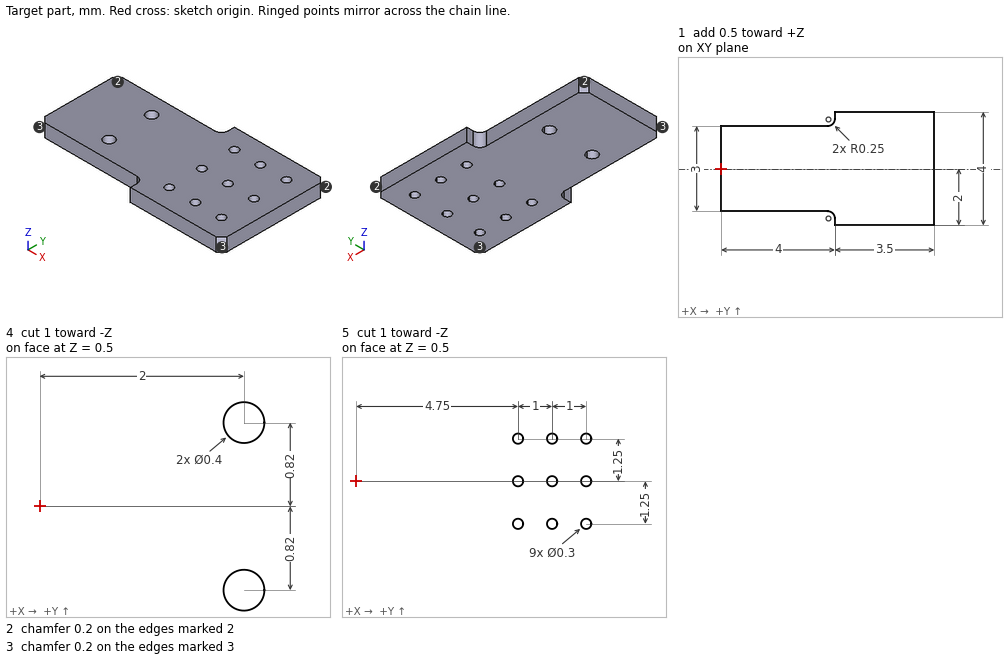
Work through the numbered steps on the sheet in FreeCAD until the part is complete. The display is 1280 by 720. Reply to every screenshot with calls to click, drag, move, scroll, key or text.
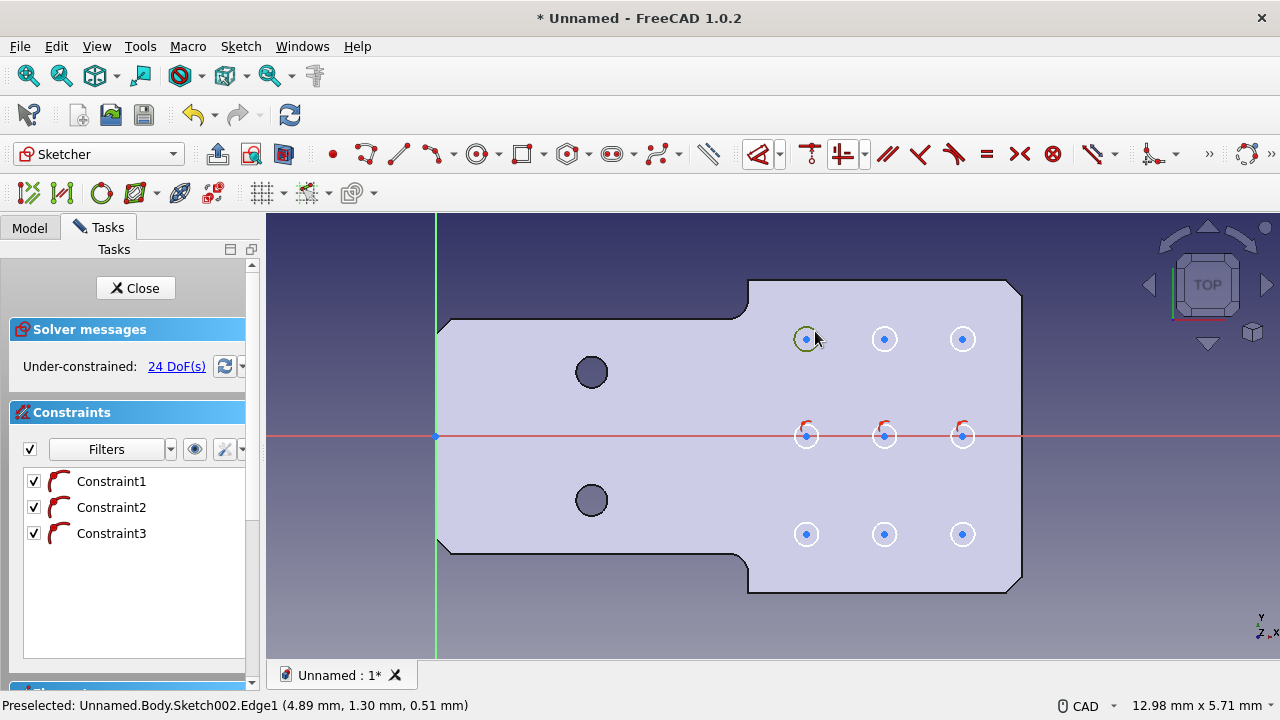
click(893, 331)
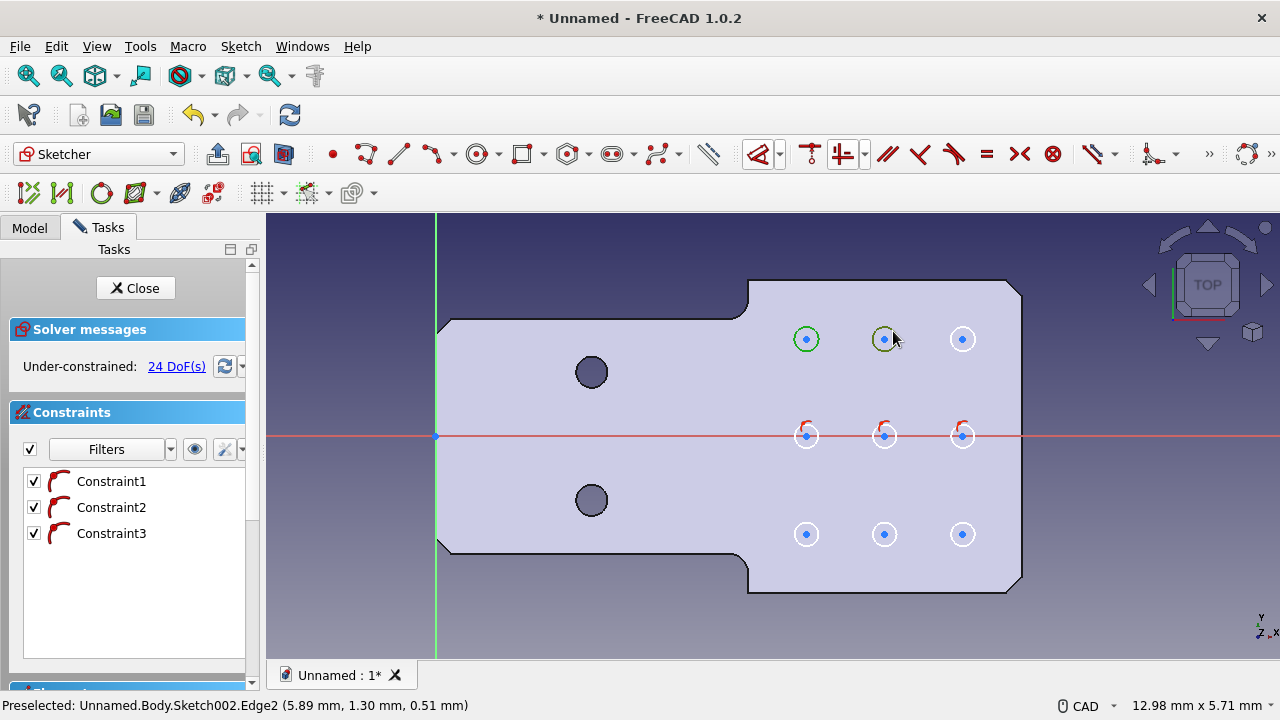
click(971, 331)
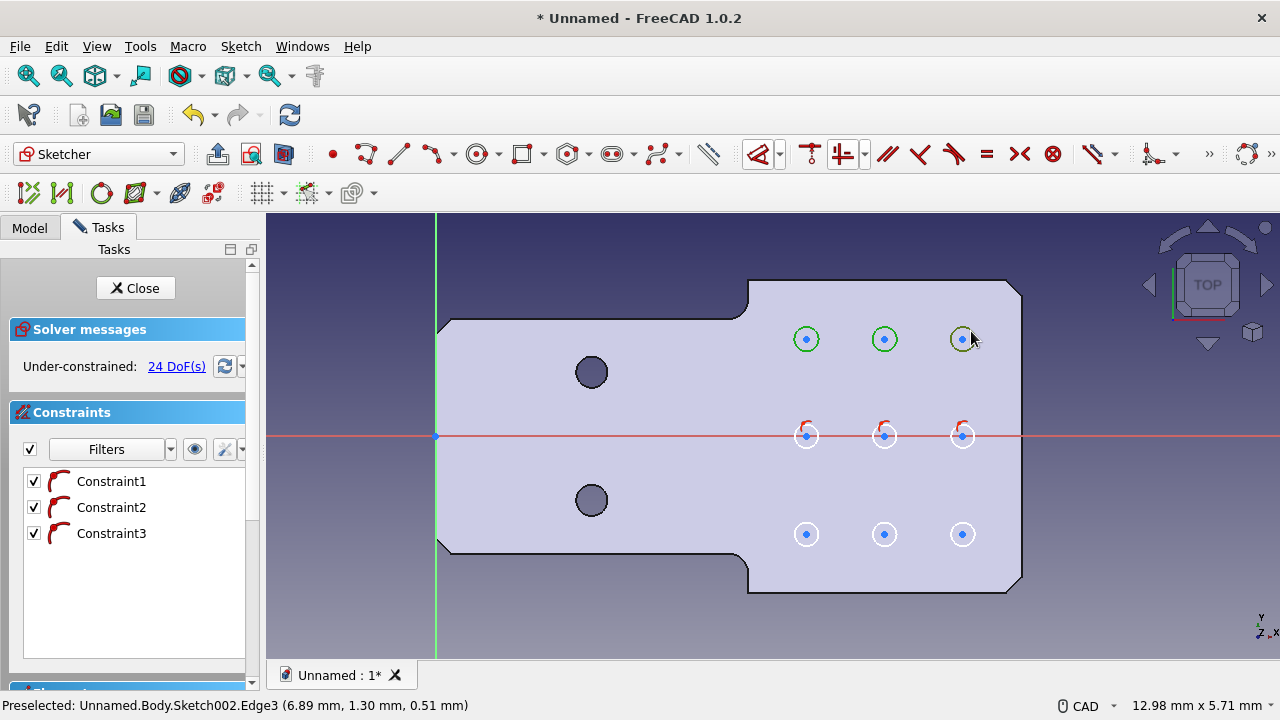
click(951, 436)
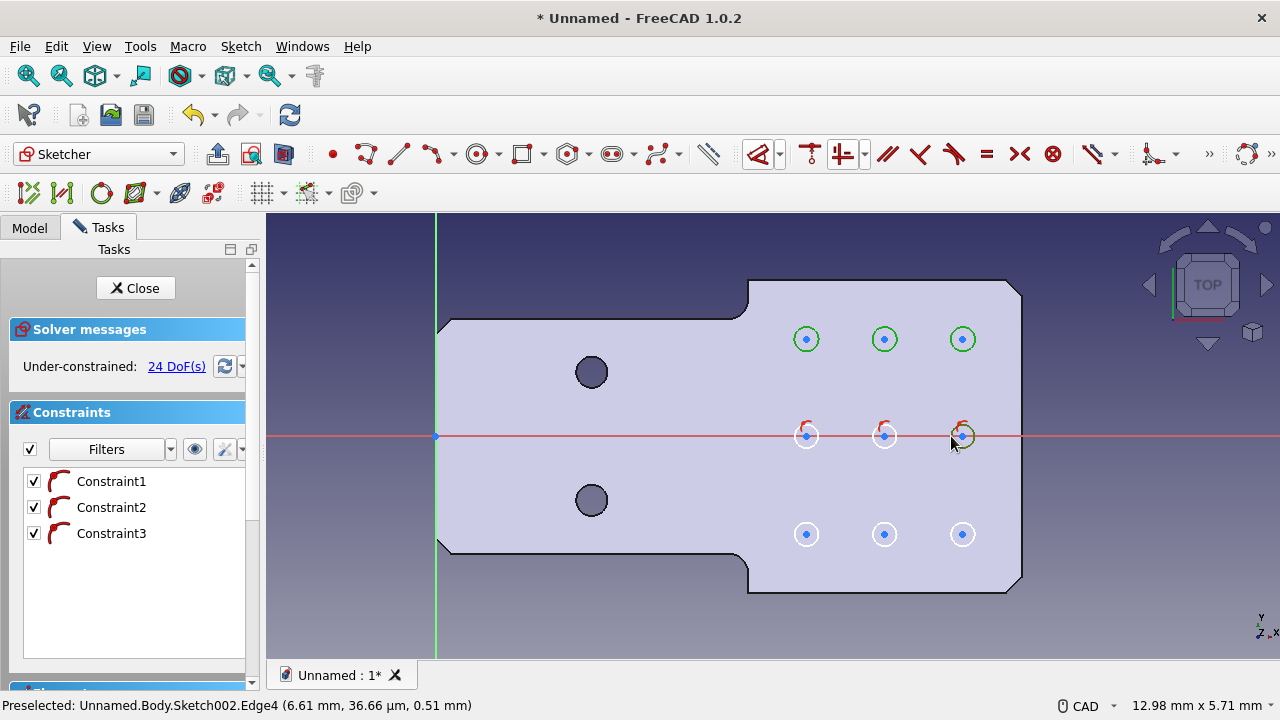
click(971, 526)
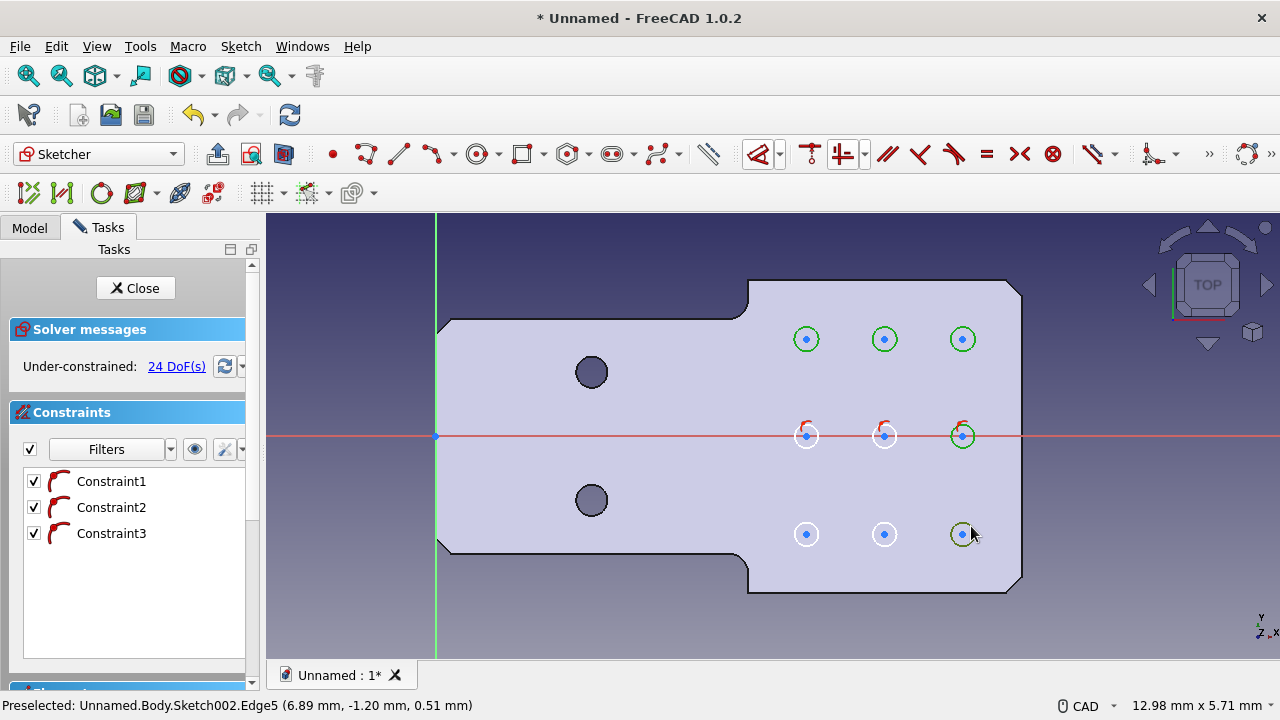
click(893, 526)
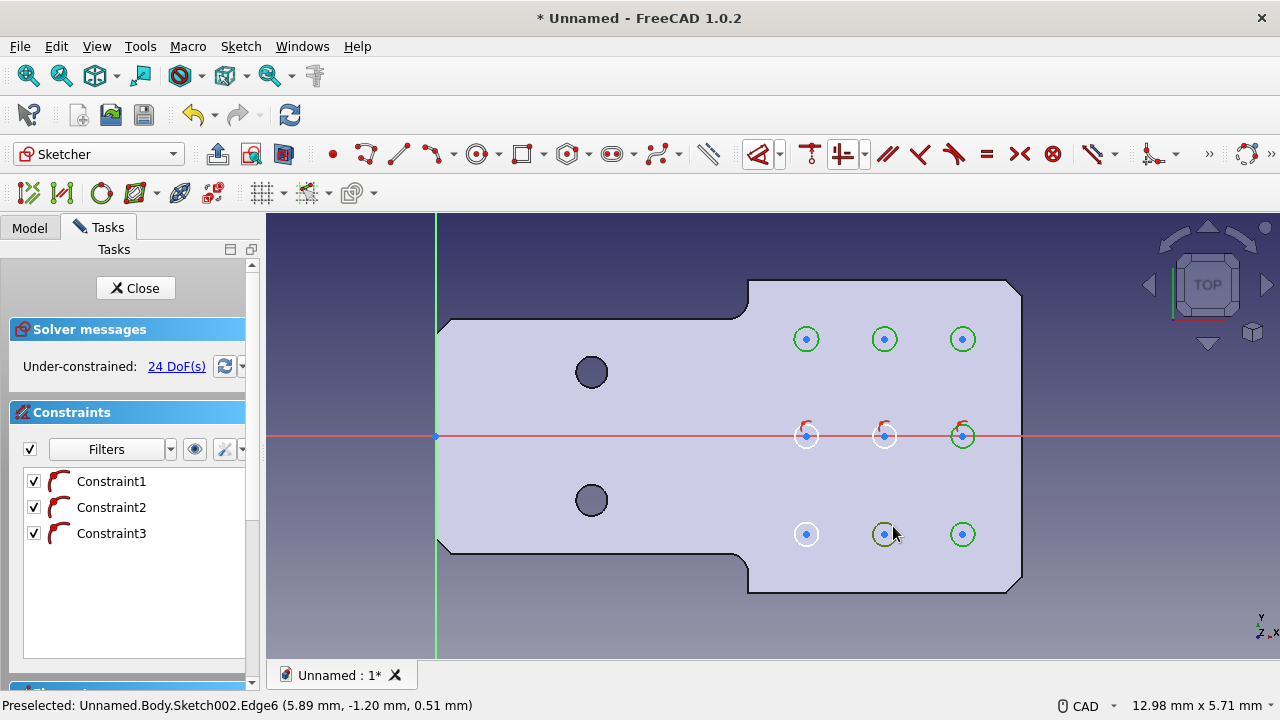
click(815, 526)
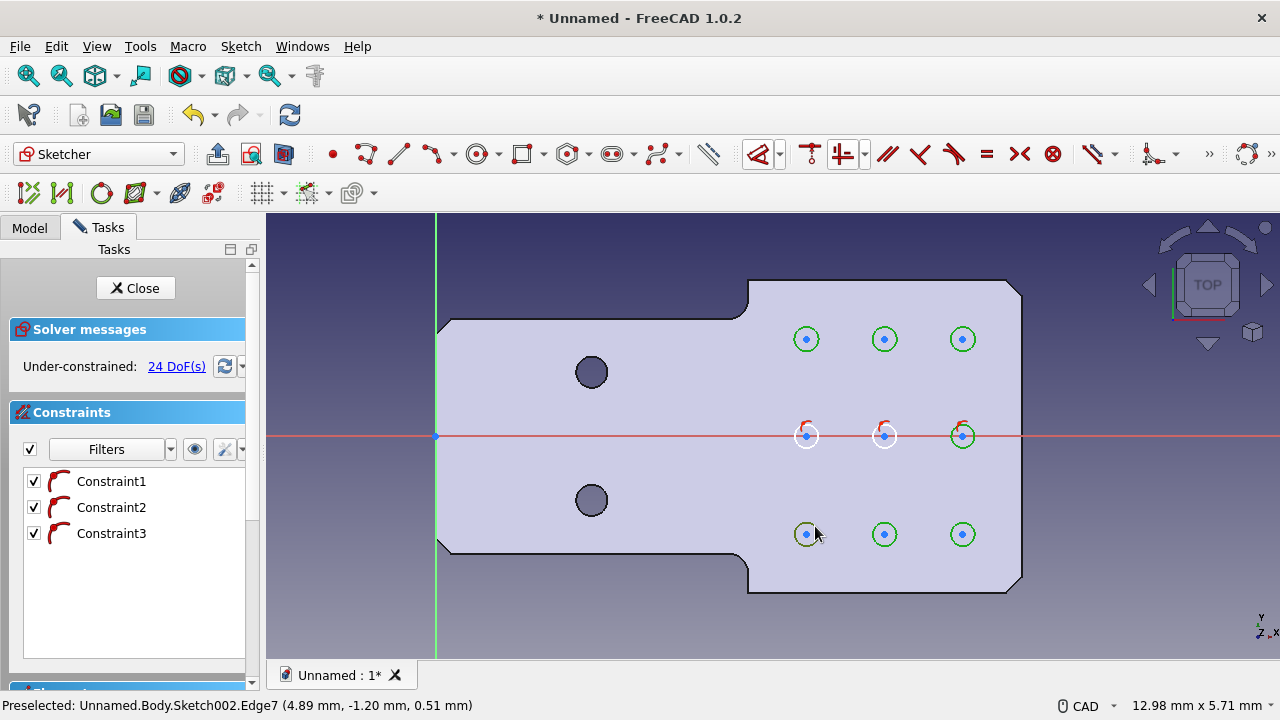
click(795, 436)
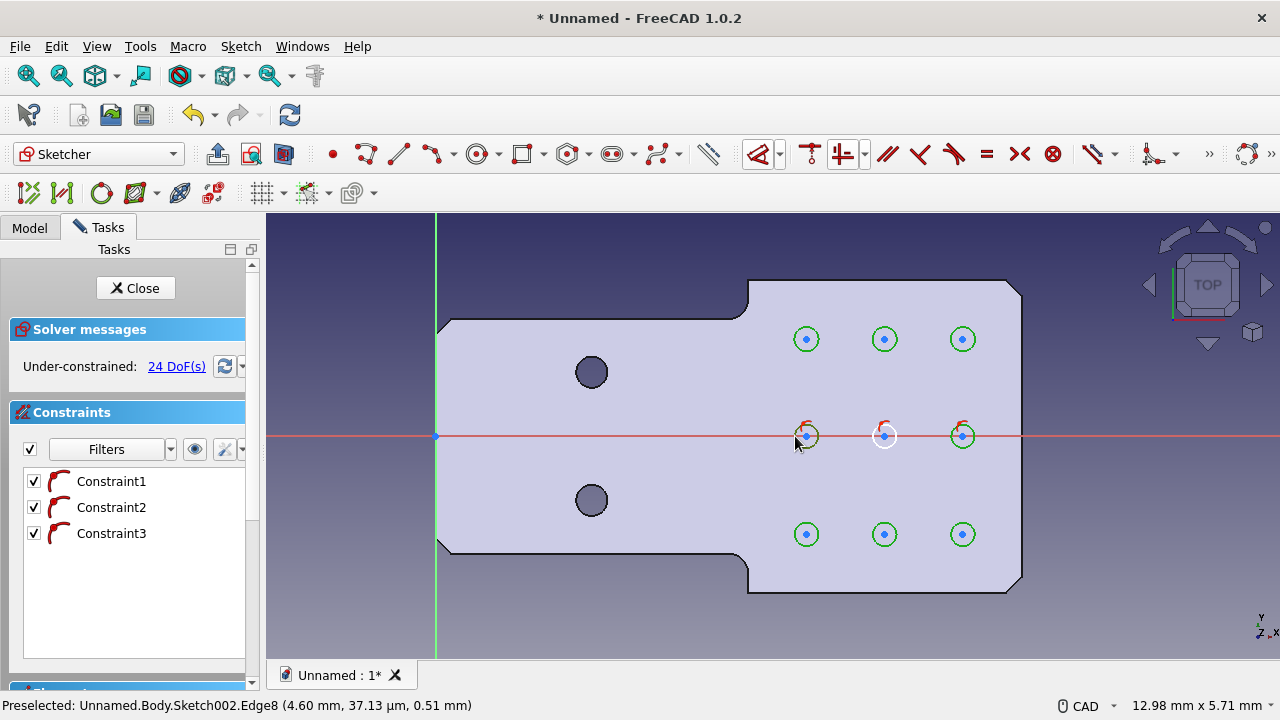
click(873, 436)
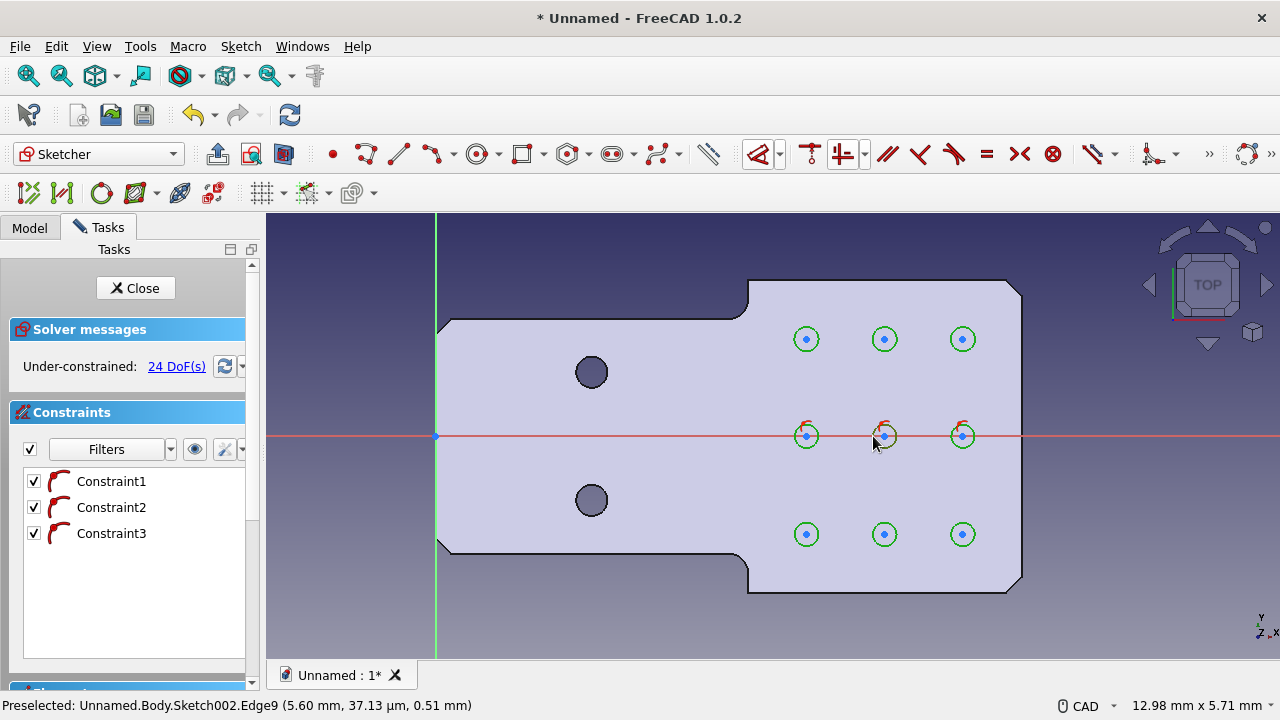
key(e)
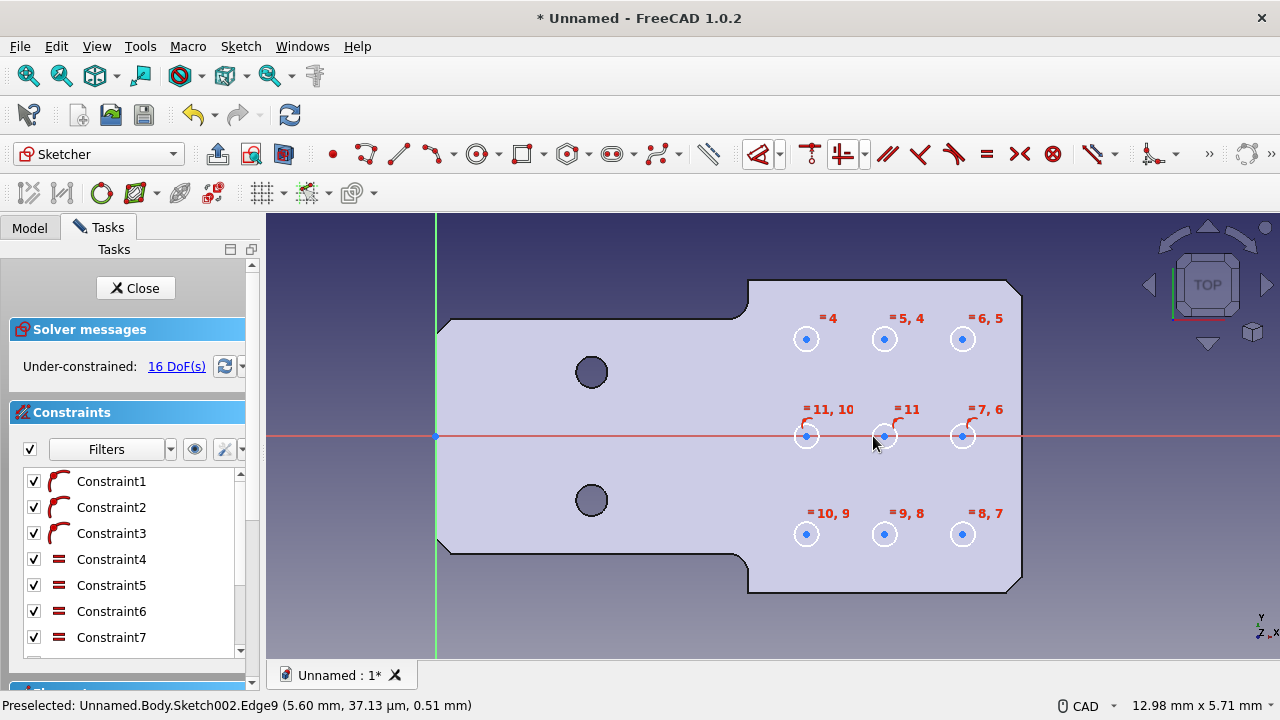
click(806, 339)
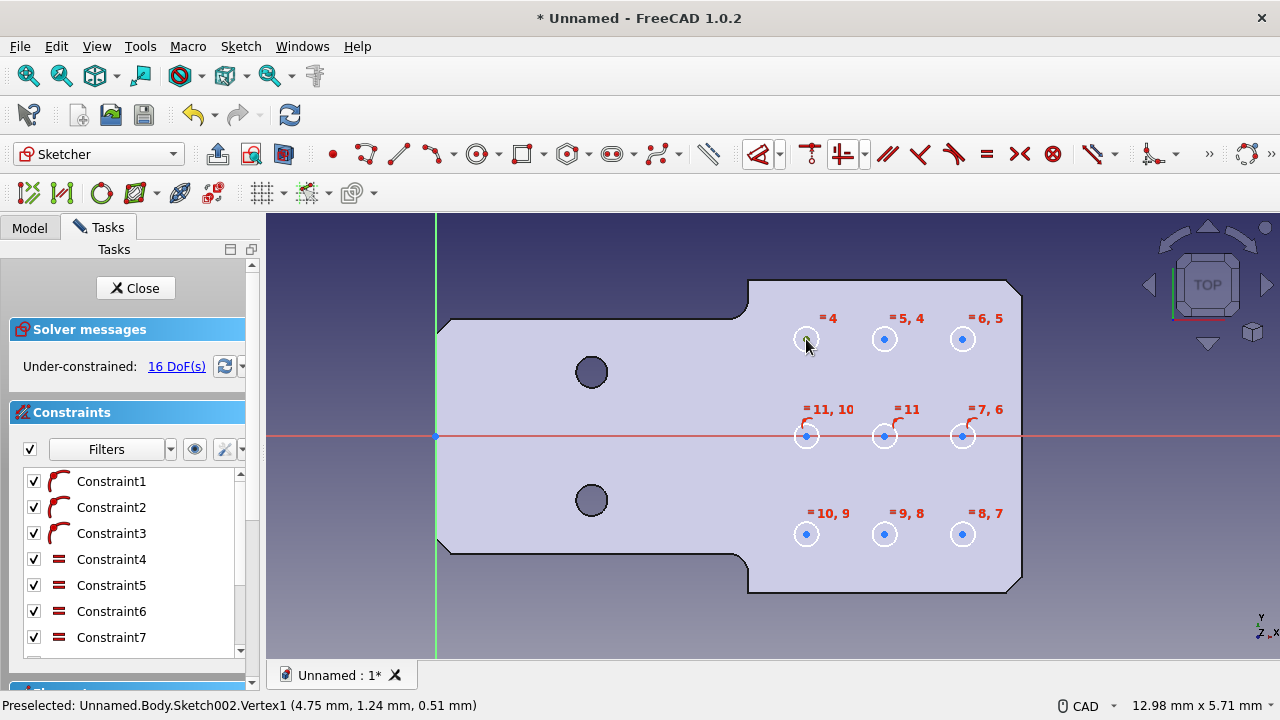
click(885, 339)